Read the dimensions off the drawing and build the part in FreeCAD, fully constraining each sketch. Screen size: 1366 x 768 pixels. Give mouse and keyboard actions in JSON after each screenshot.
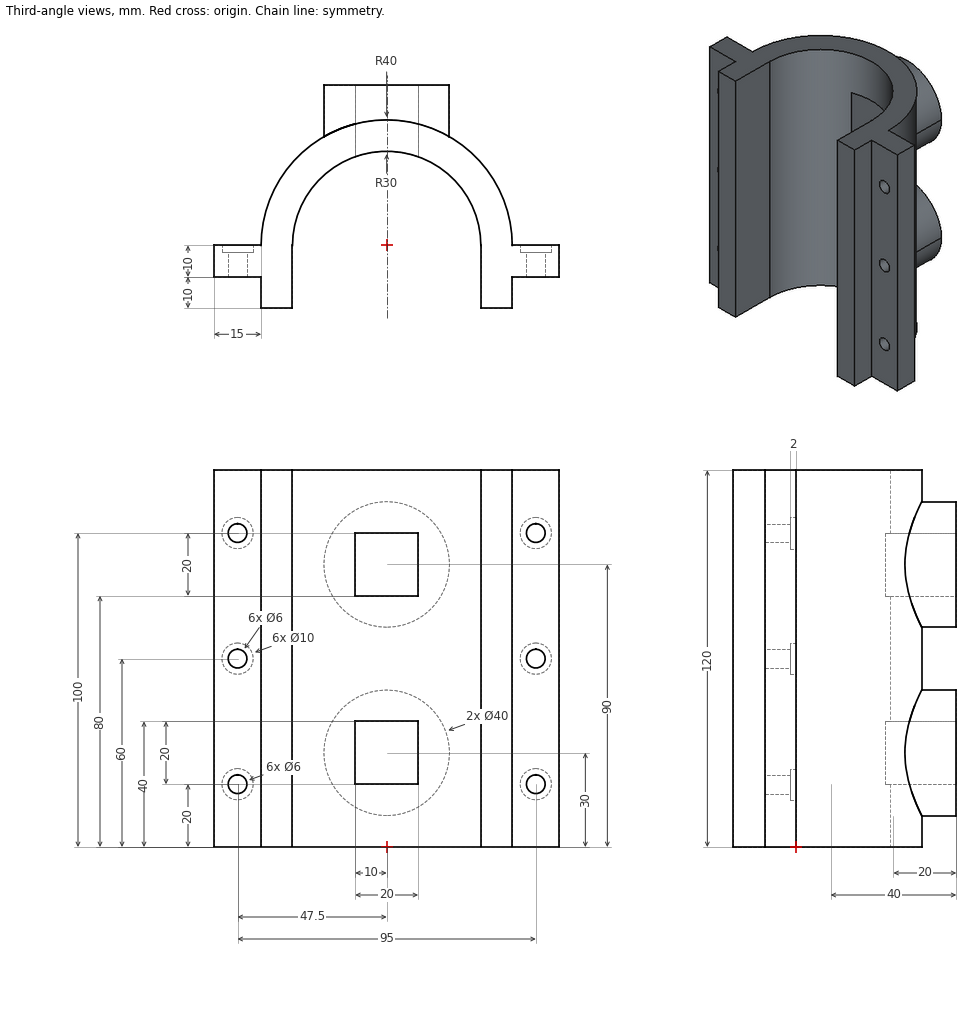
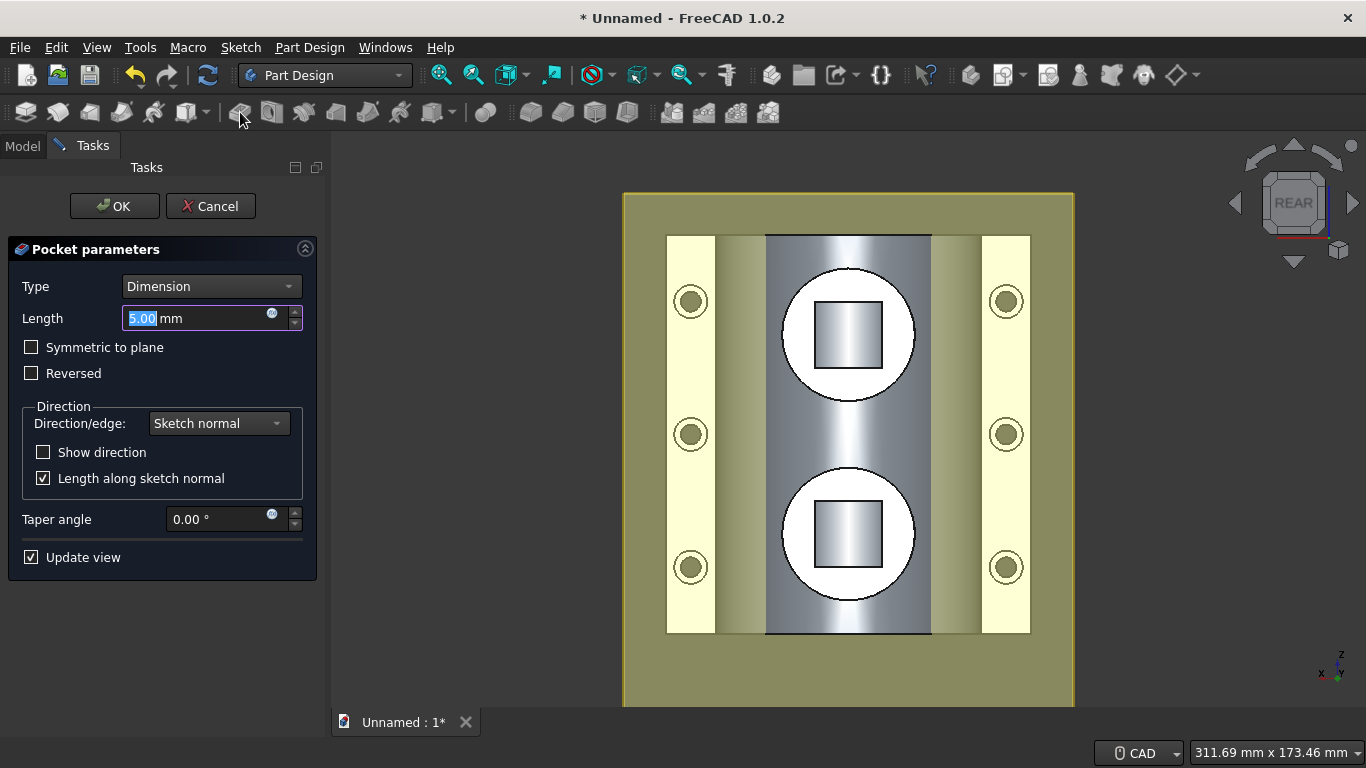
{"action": "type", "text": "40"}
{"action": "key", "text": "Tab"}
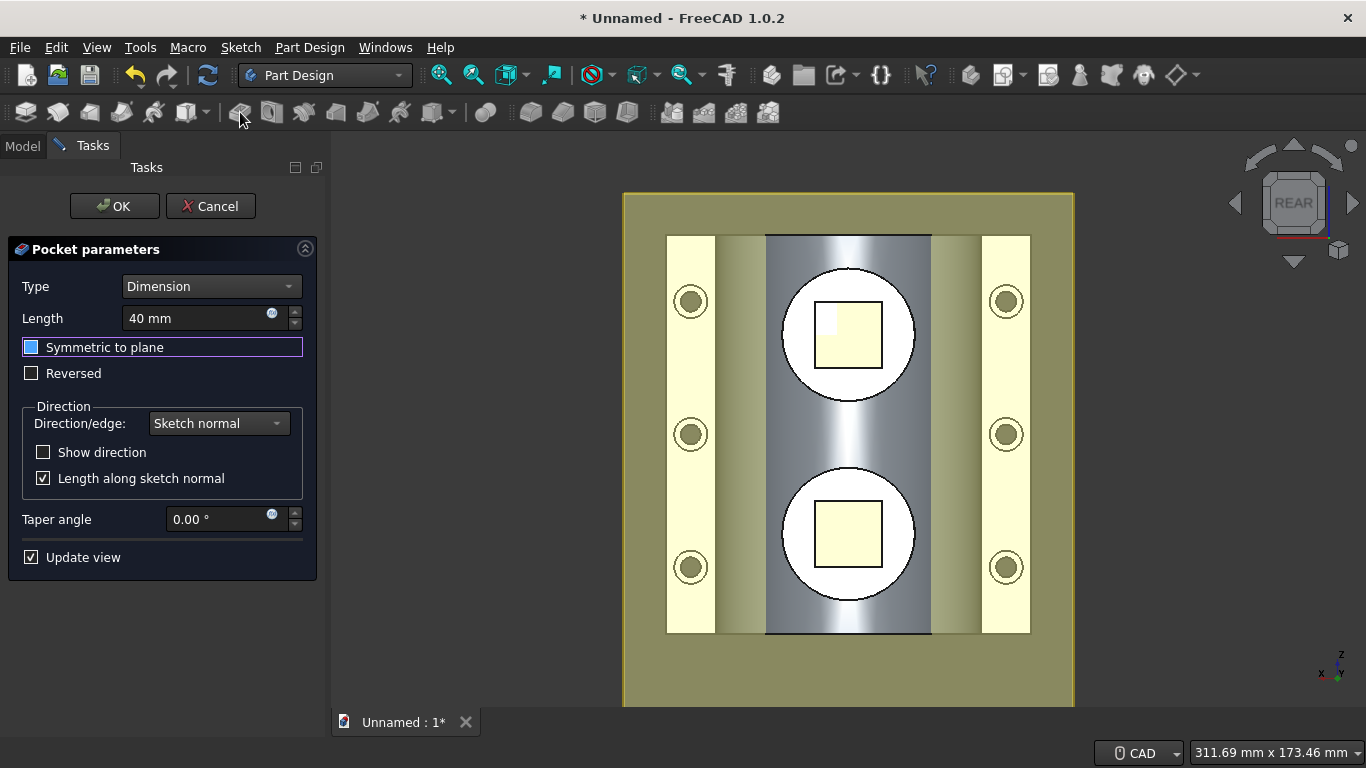
{"action": "left_click", "coordinate": [30, 347]}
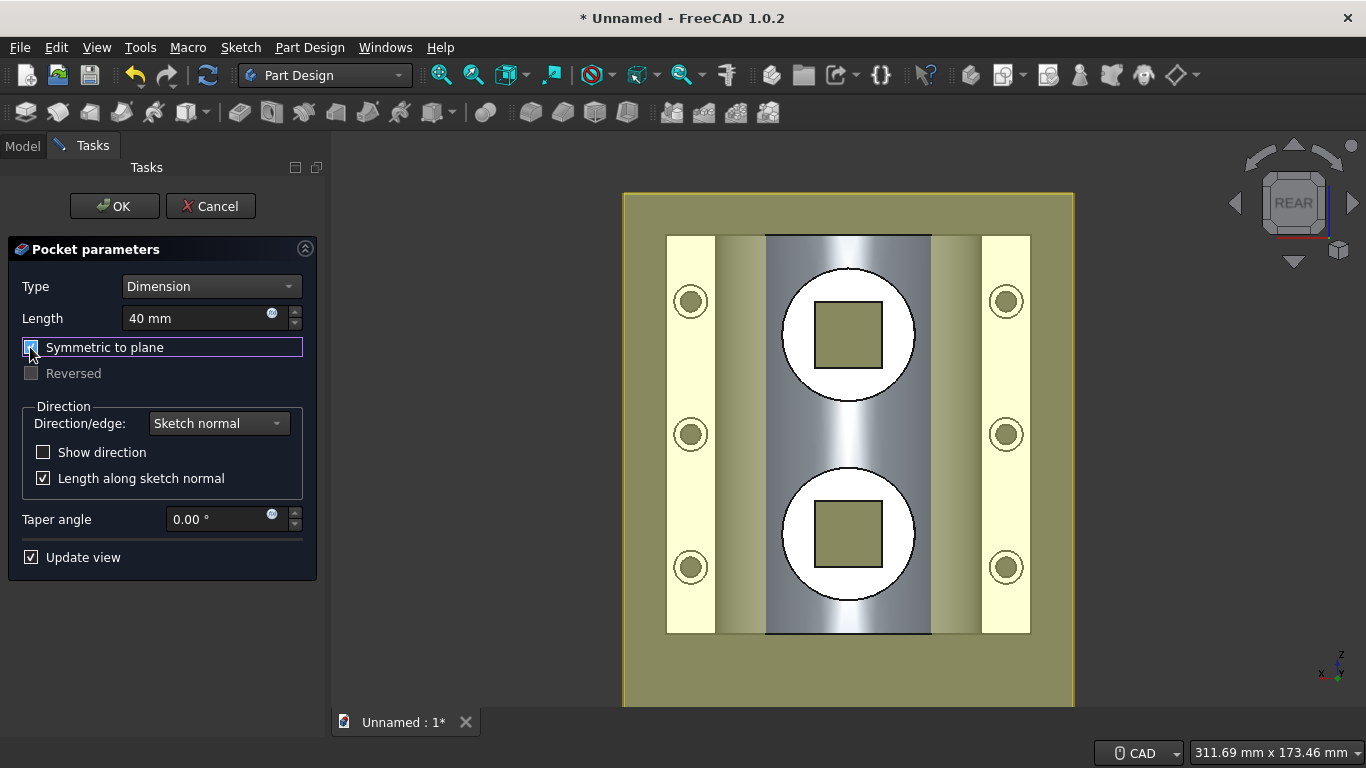
{"action": "left_click", "coordinate": [115, 206]}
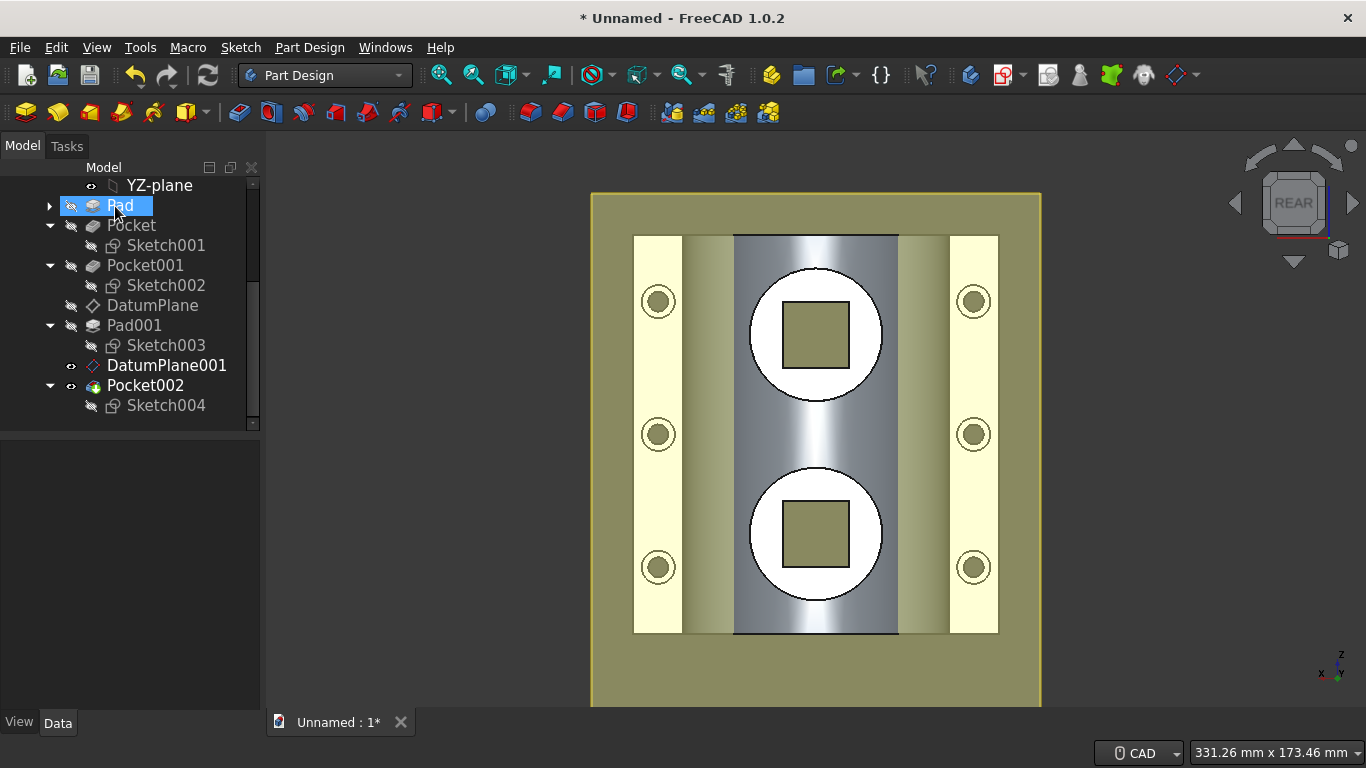
{"action": "left_click", "coordinate": [116, 366]}
{"action": "key", "text": "space"}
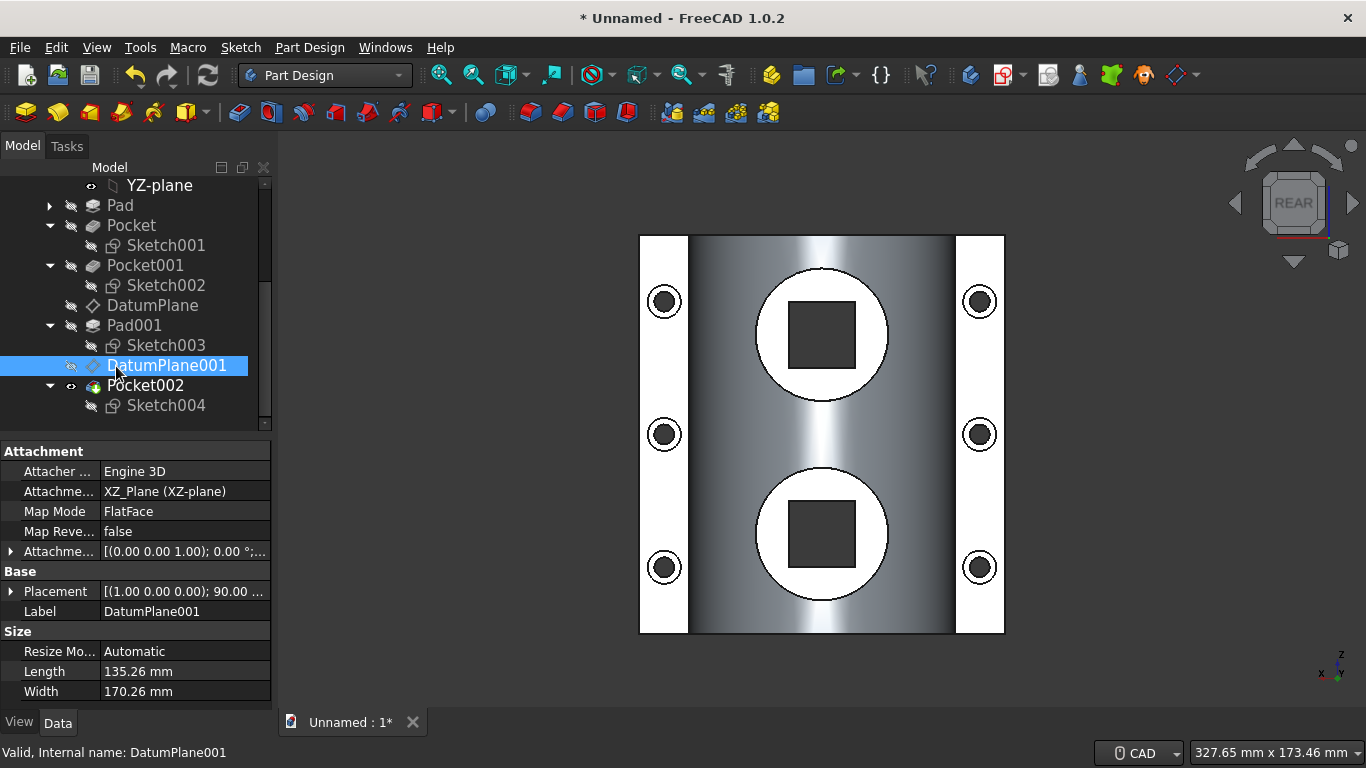
{"action": "key", "text": "0"}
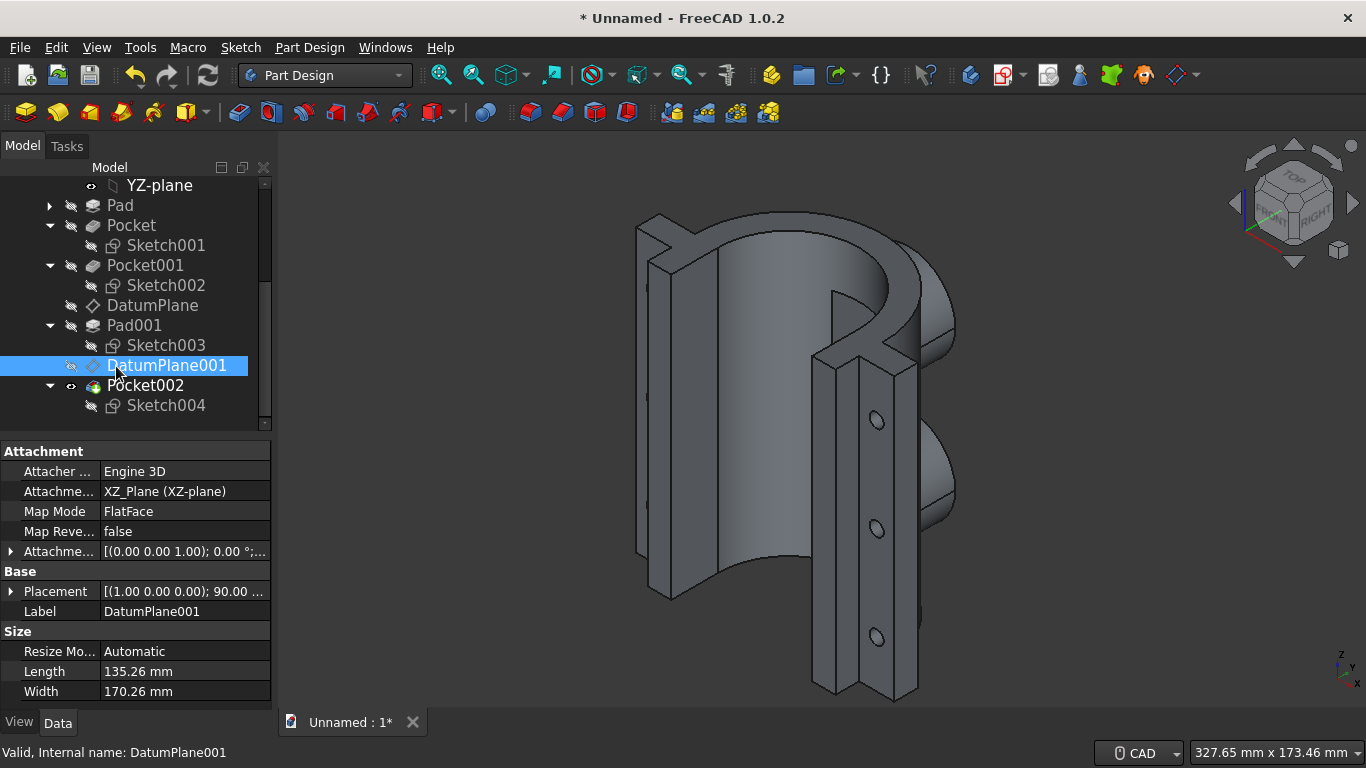
{"action": "left_click", "coordinate": [442, 76]}